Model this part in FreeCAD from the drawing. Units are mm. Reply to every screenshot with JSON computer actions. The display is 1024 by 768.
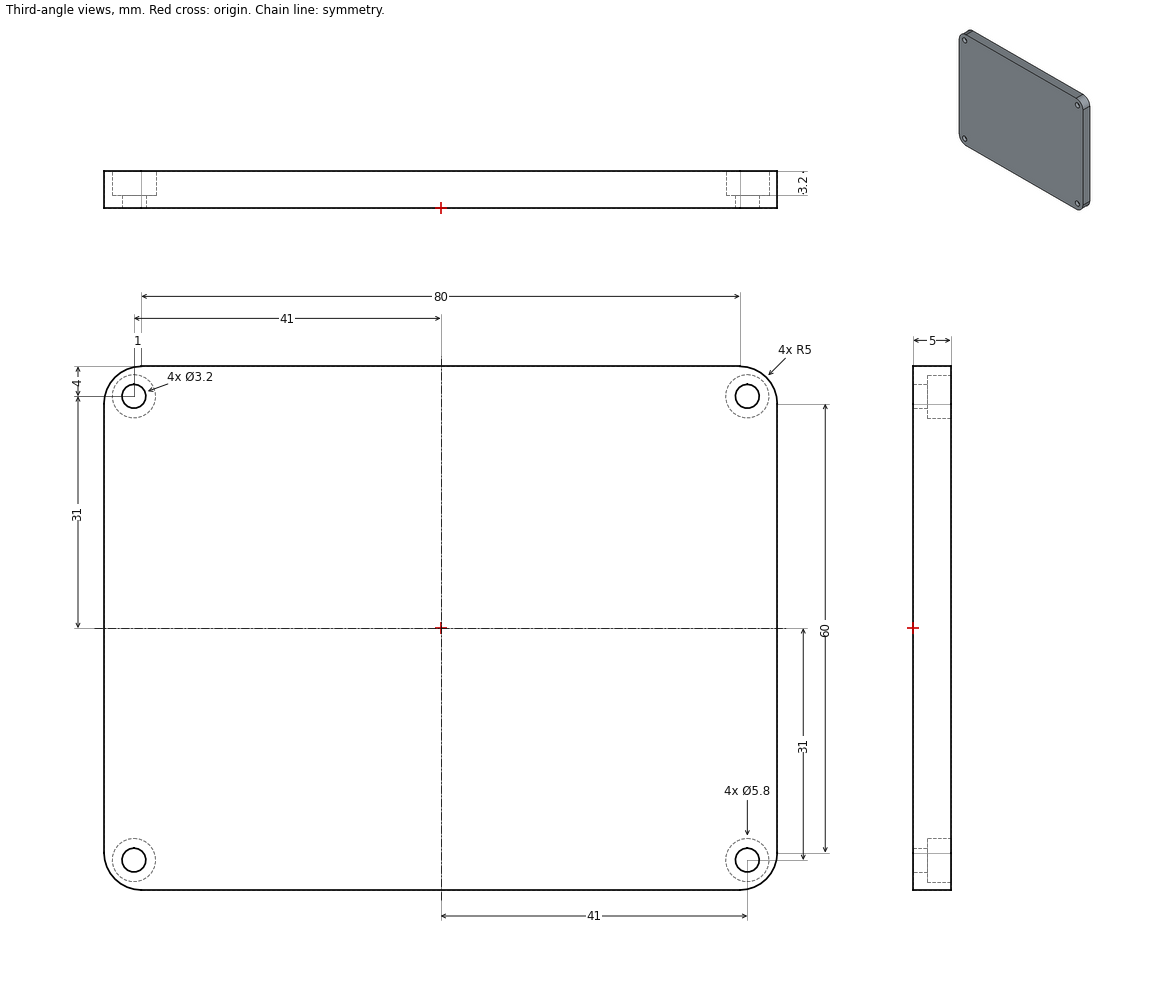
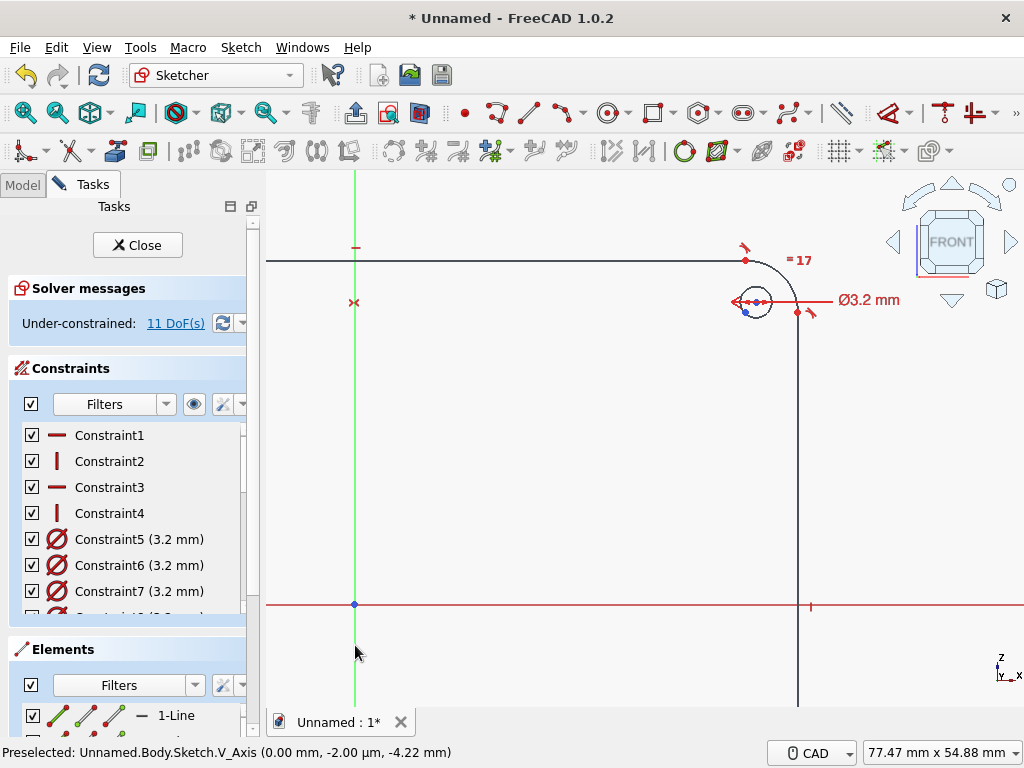
{"action": "scroll", "coordinate": [757, 303], "scroll_direction": "down", "scroll_amount": 4}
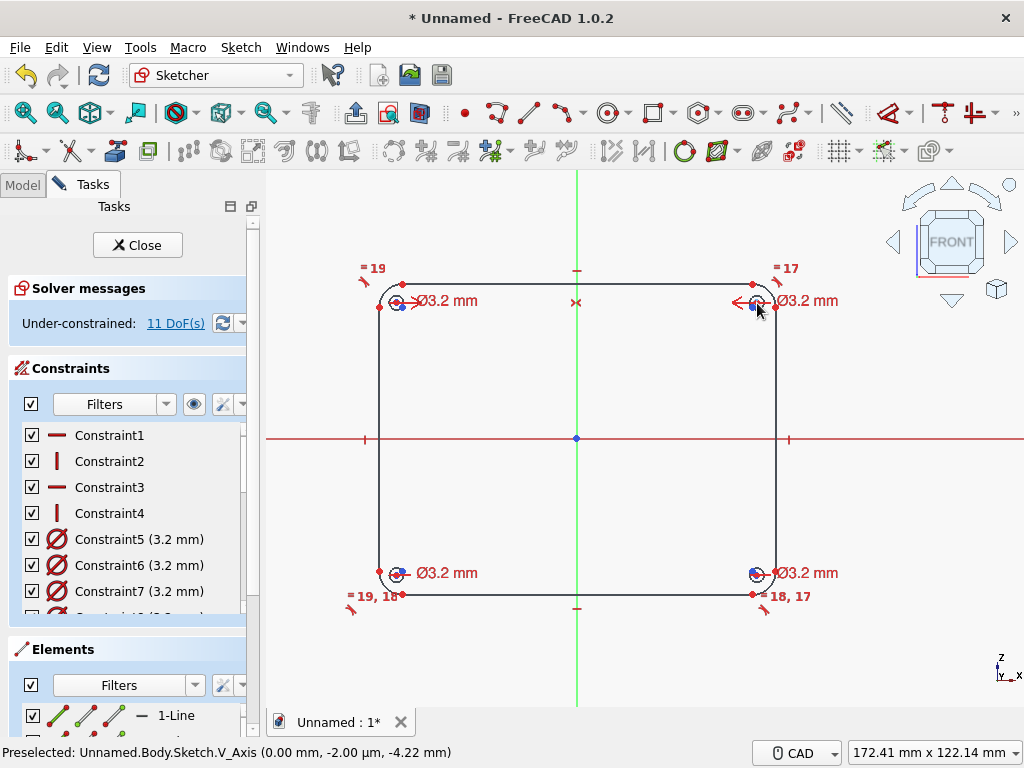
{"action": "scroll", "coordinate": [396, 303], "scroll_direction": "up", "scroll_amount": 3}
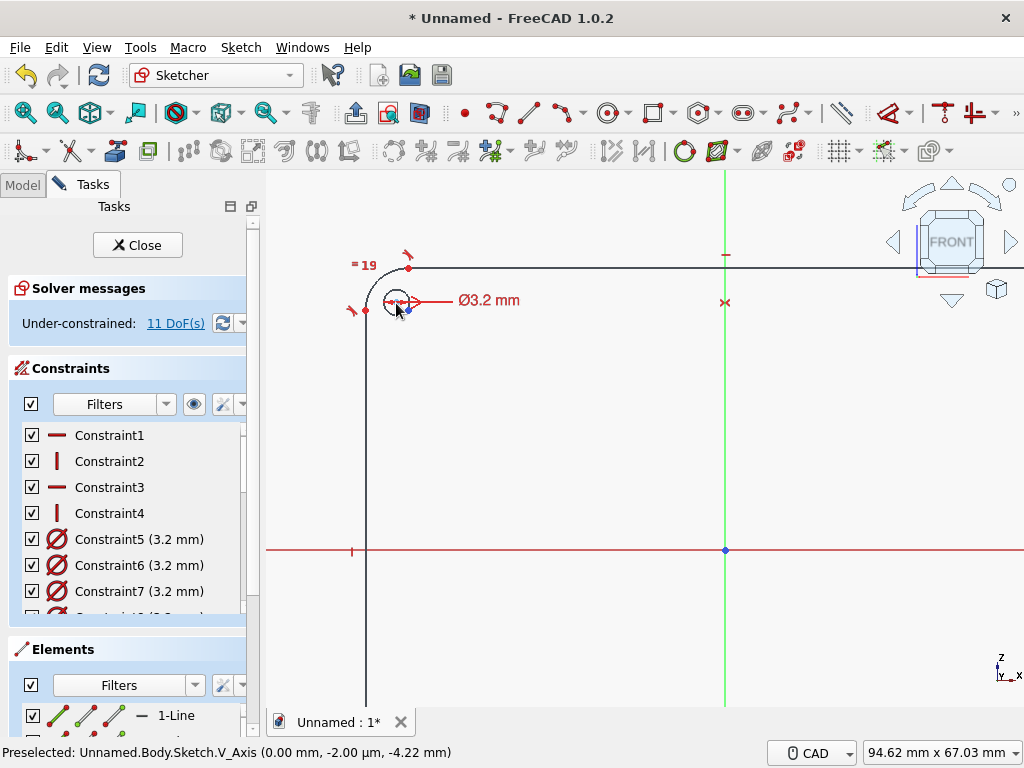
{"action": "left_click", "coordinate": [397, 302]}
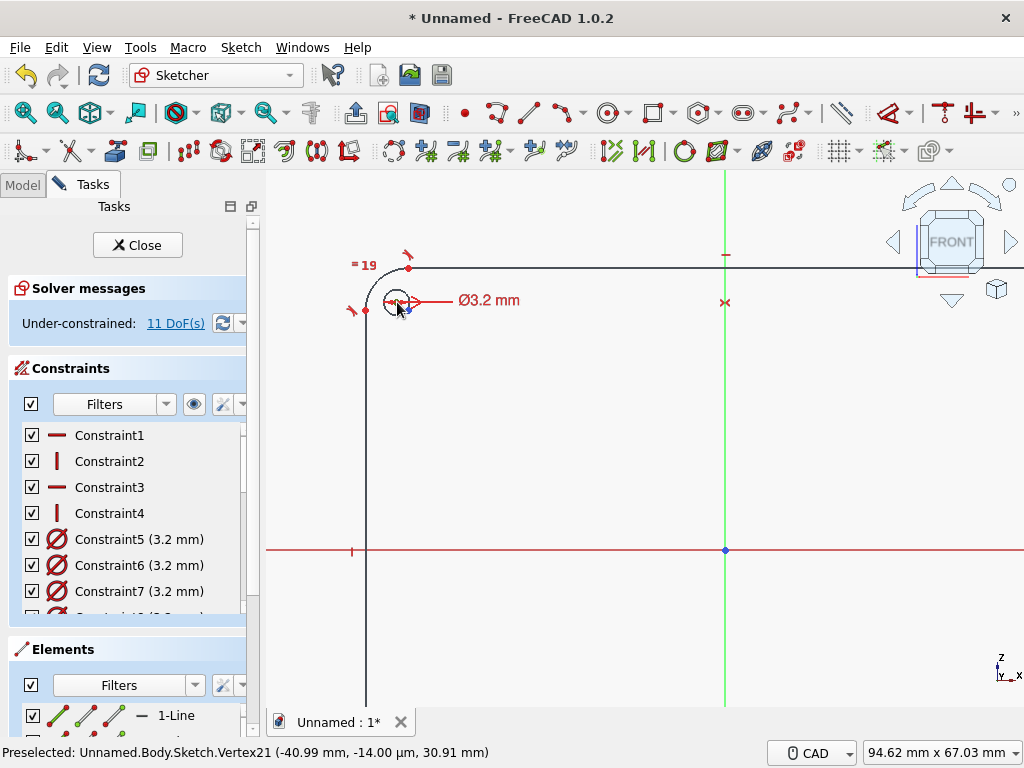
{"action": "scroll", "coordinate": [396, 303], "scroll_direction": "down", "scroll_amount": 3}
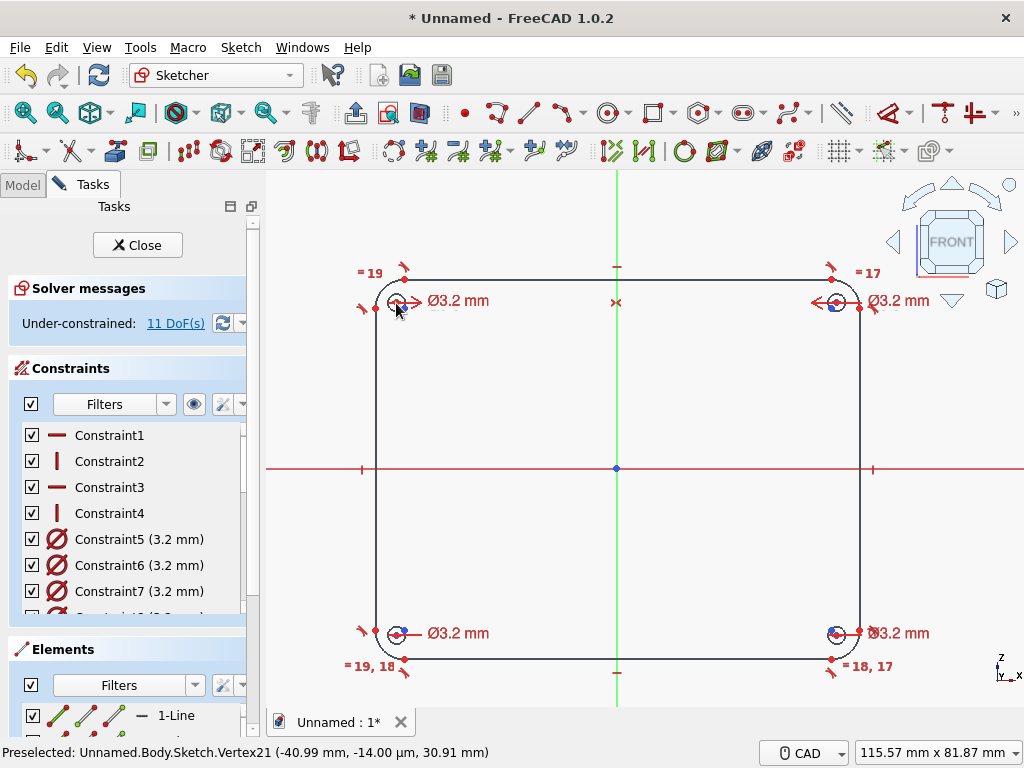
{"action": "scroll", "coordinate": [396, 575], "scroll_direction": "up", "scroll_amount": 3}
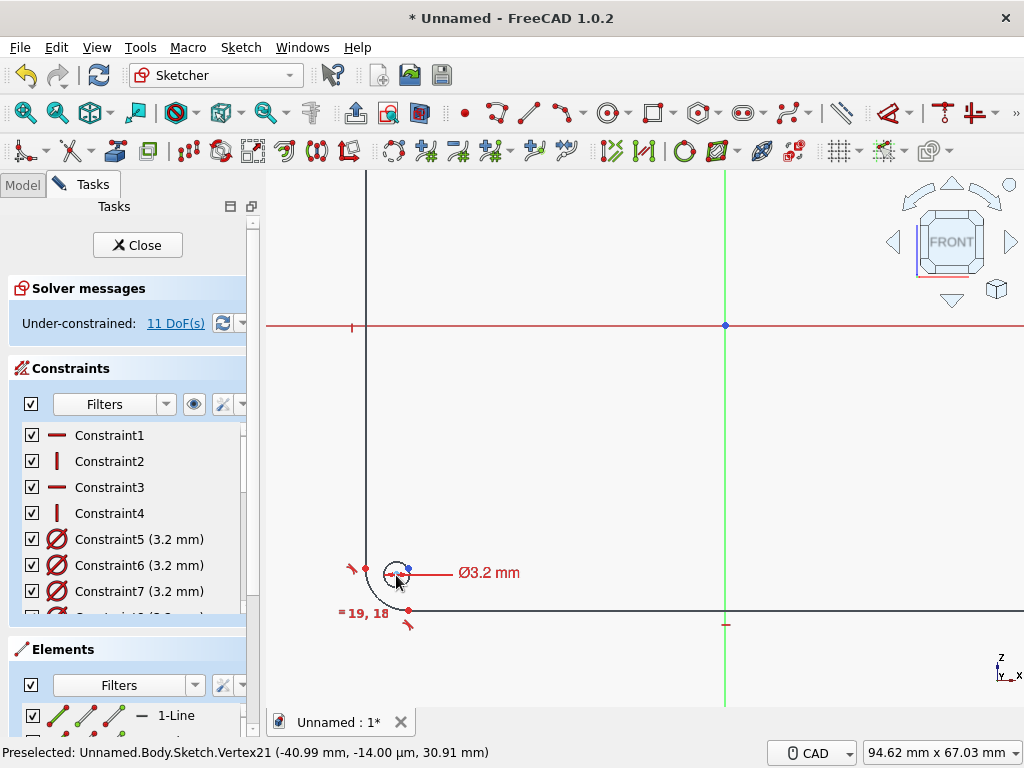
{"action": "left_click", "coordinate": [397, 575]}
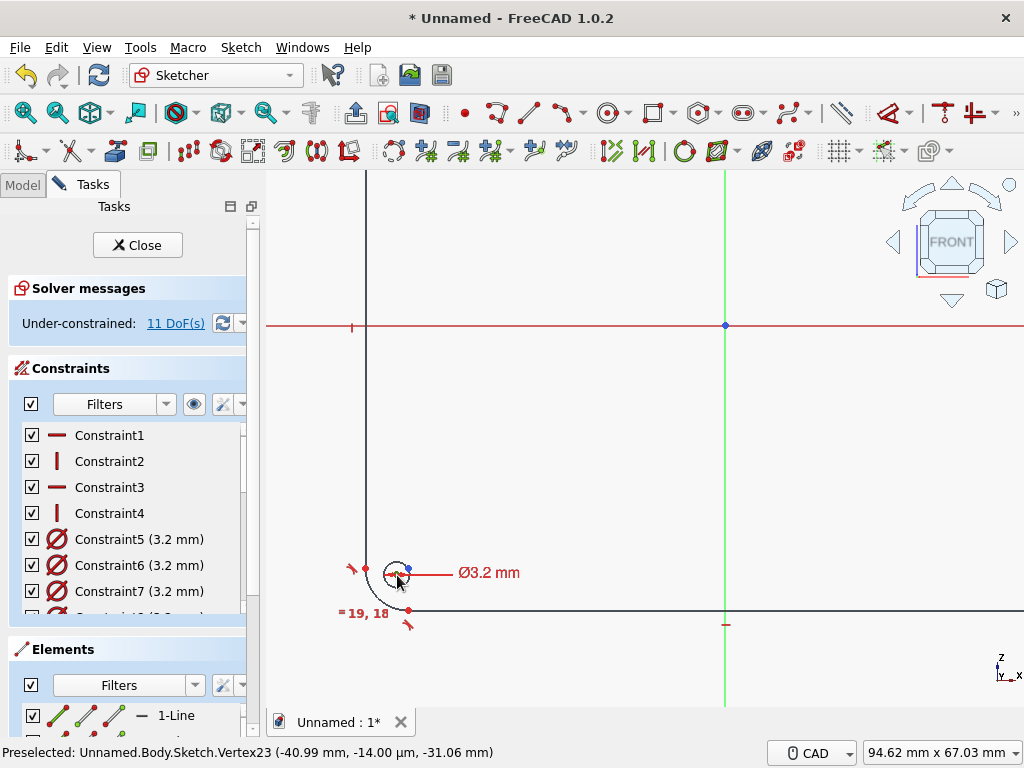
{"action": "left_click", "coordinate": [334, 326]}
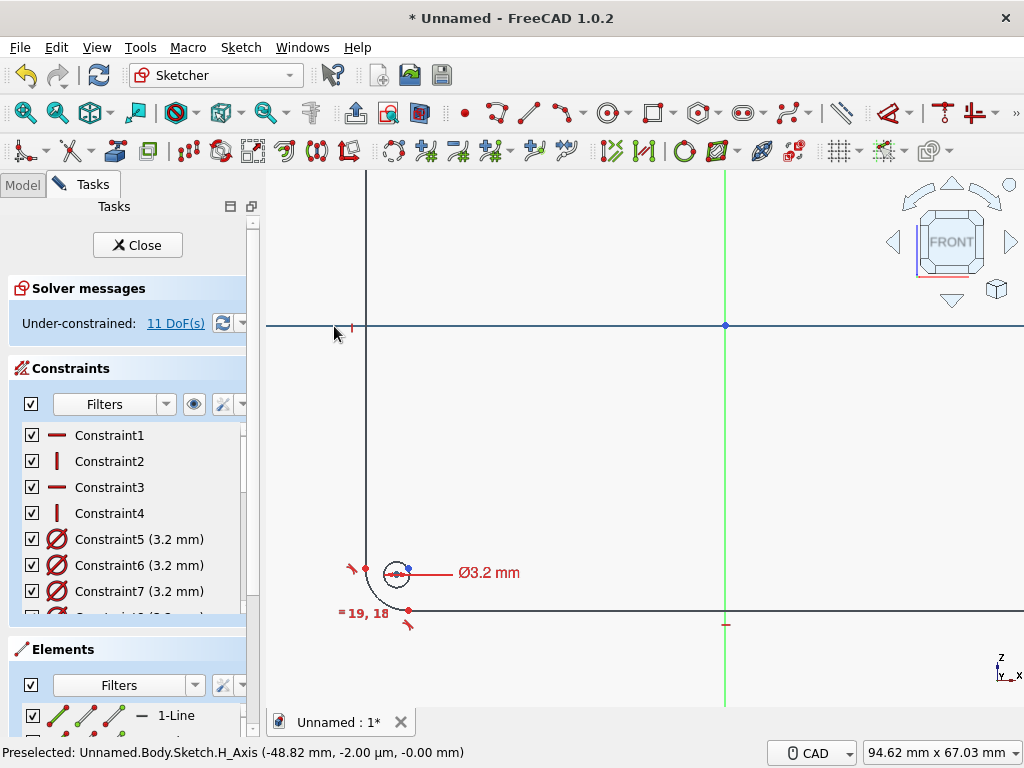
{"action": "key", "text": "s"}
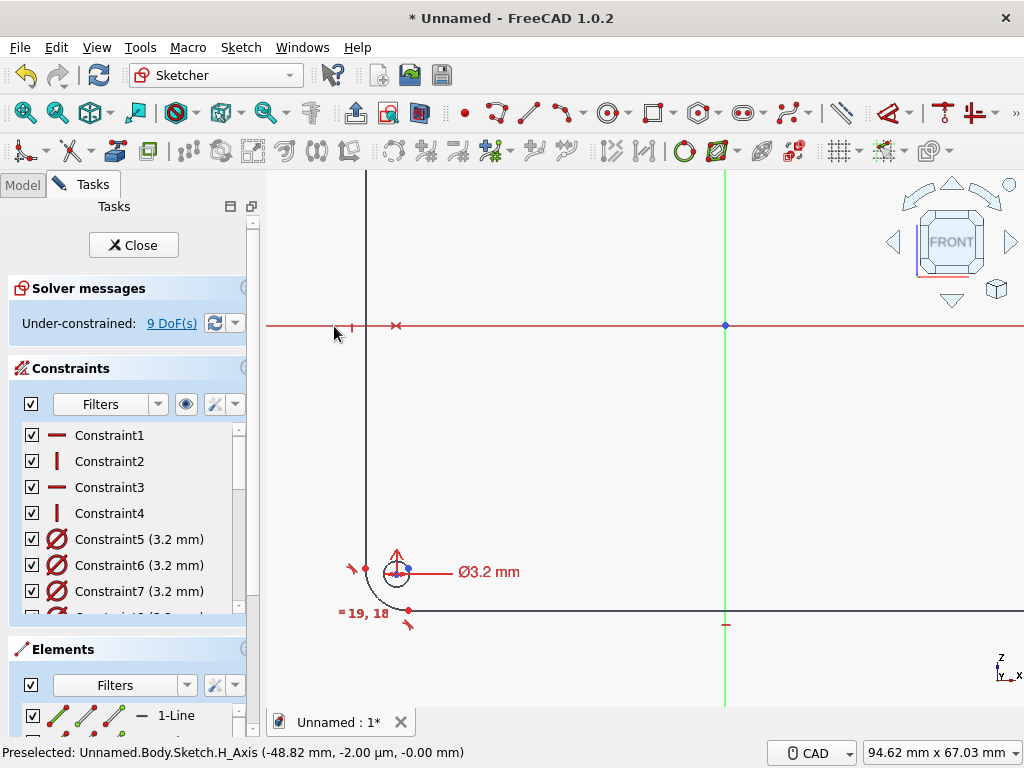
{"action": "scroll", "coordinate": [396, 575], "scroll_direction": "down", "scroll_amount": 3}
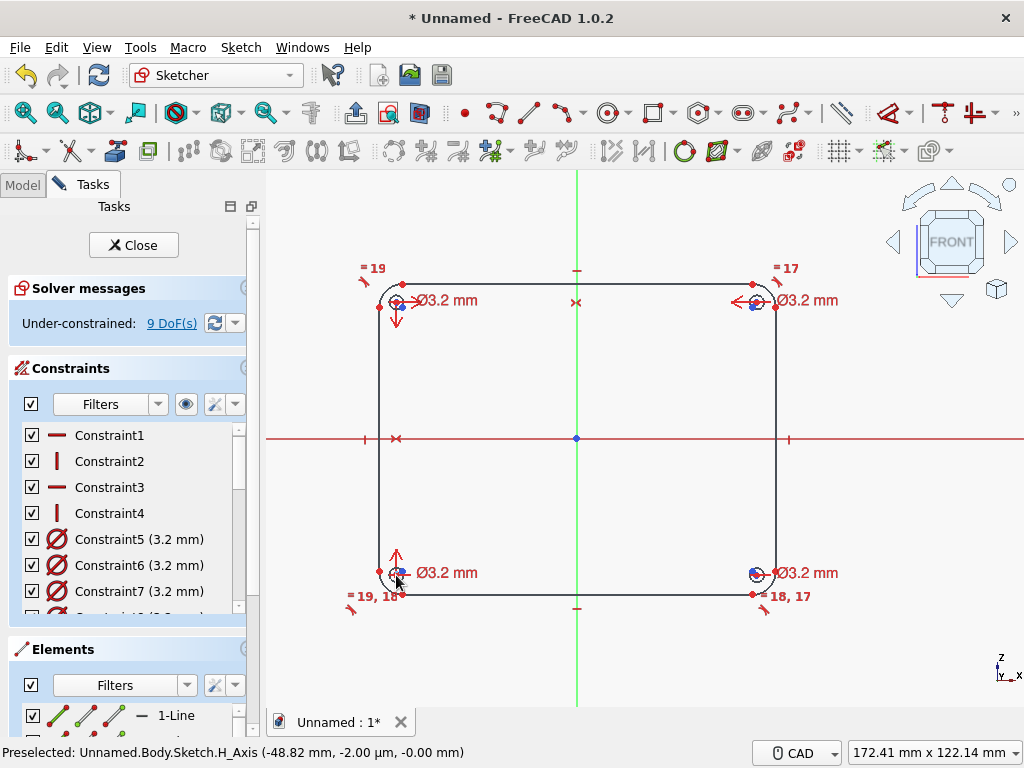
{"action": "scroll", "coordinate": [757, 302], "scroll_direction": "up", "scroll_amount": 3}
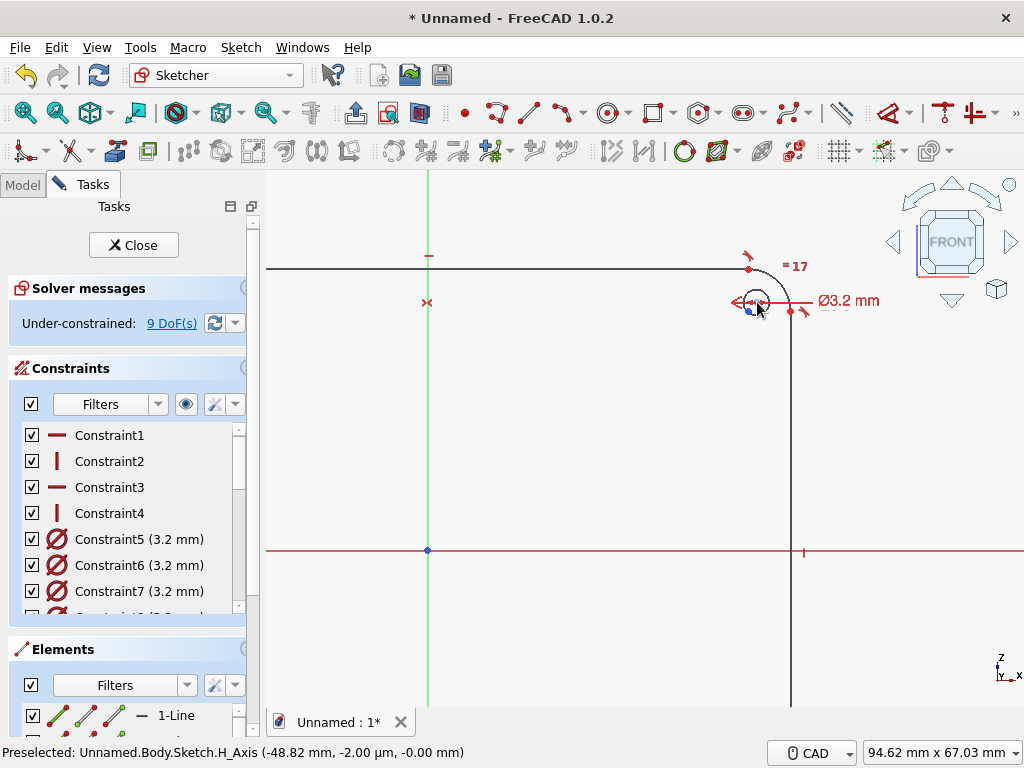
{"action": "left_click", "coordinate": [756, 303]}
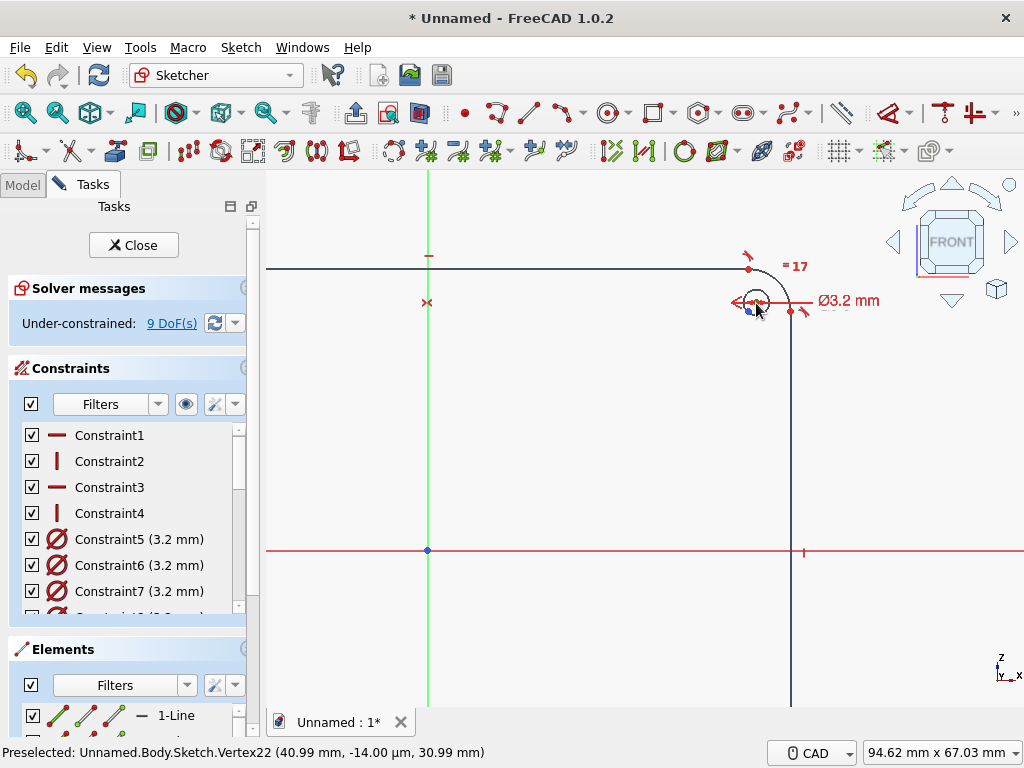
{"action": "scroll", "coordinate": [757, 302], "scroll_direction": "down", "scroll_amount": 3}